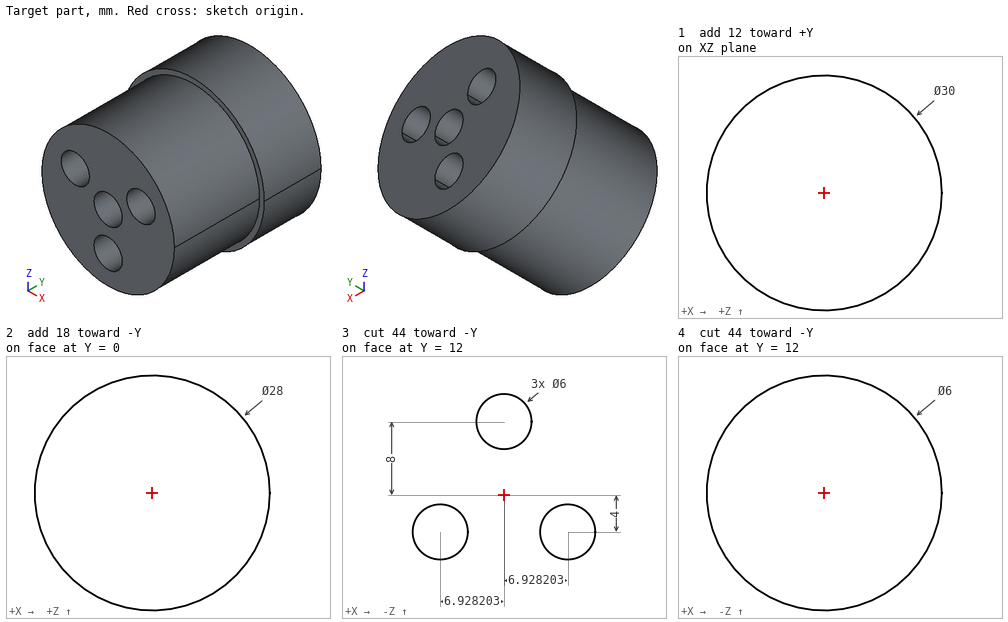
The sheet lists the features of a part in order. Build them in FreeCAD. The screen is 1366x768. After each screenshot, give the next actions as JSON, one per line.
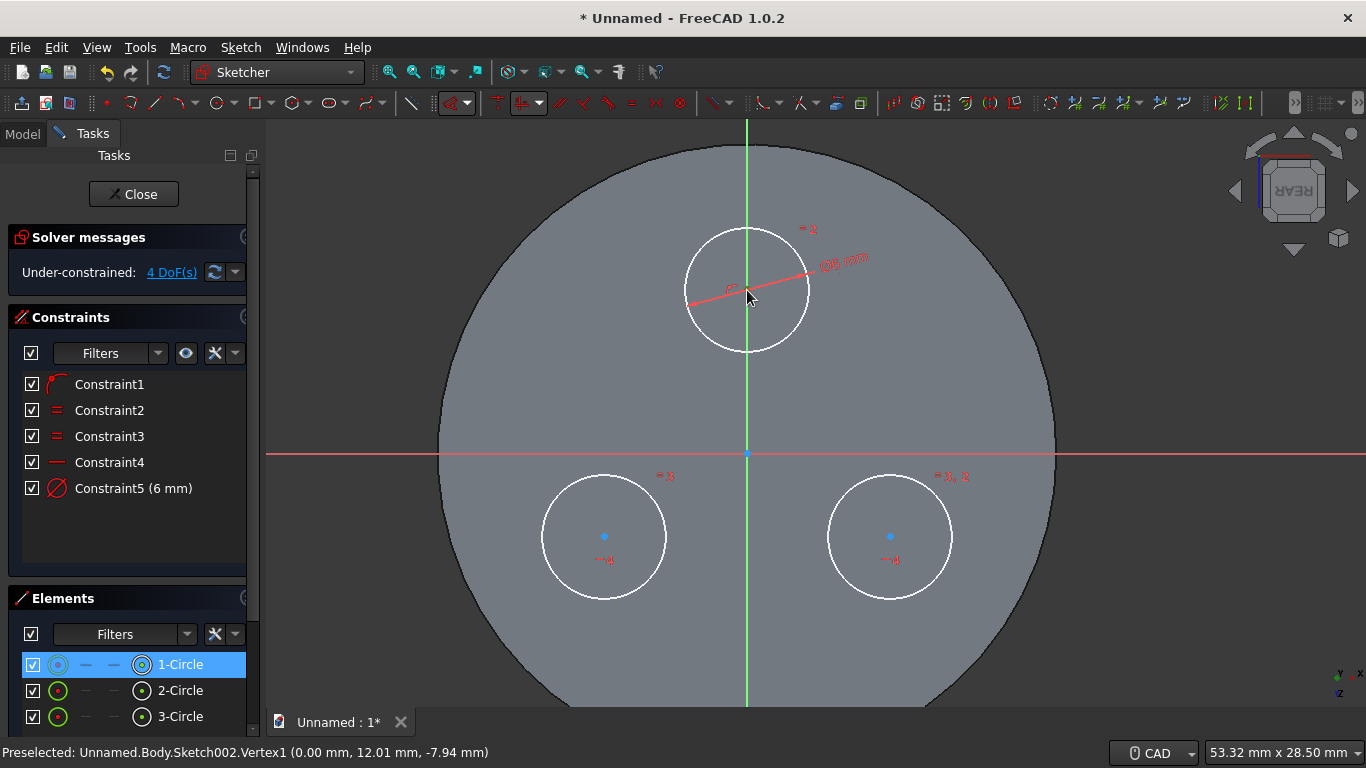
{"action": "key", "text": "i"}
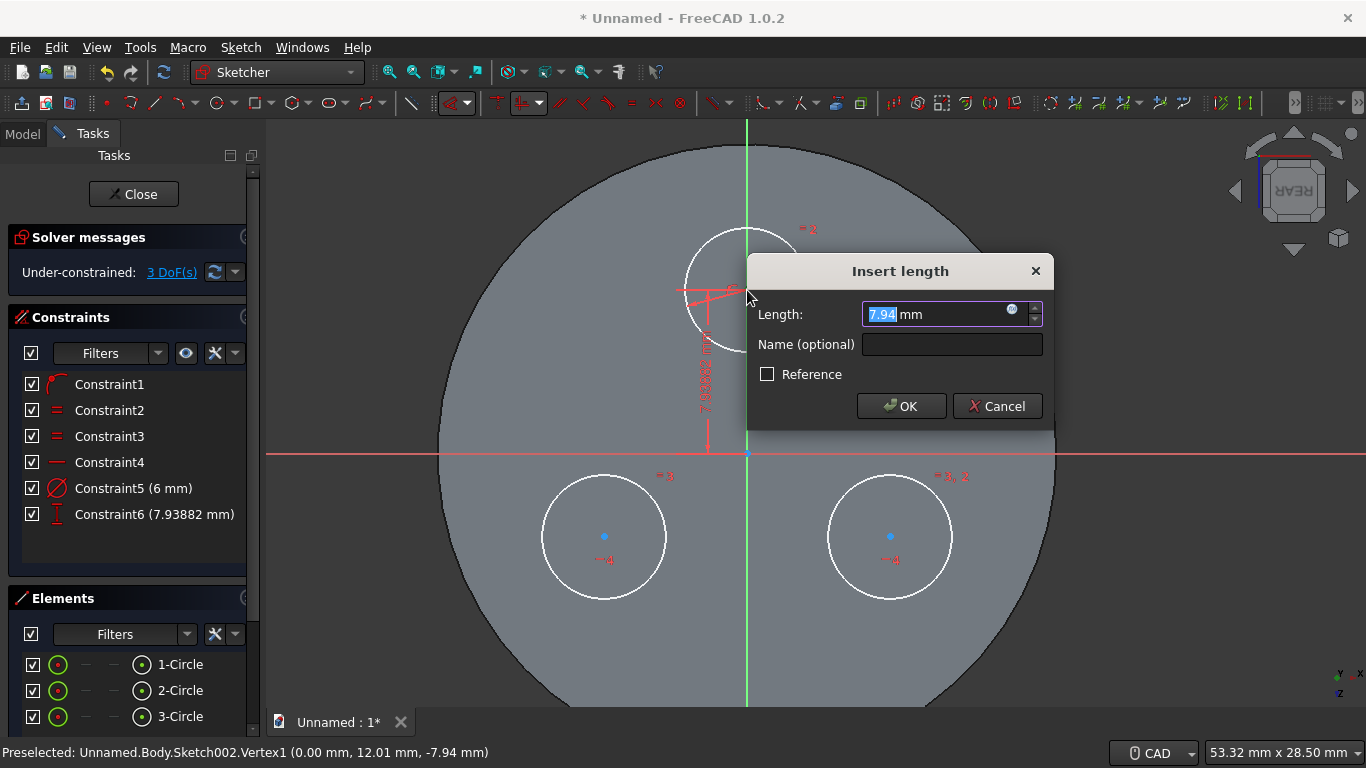
{"action": "type", "text": "8"}
{"action": "key", "text": "Return"}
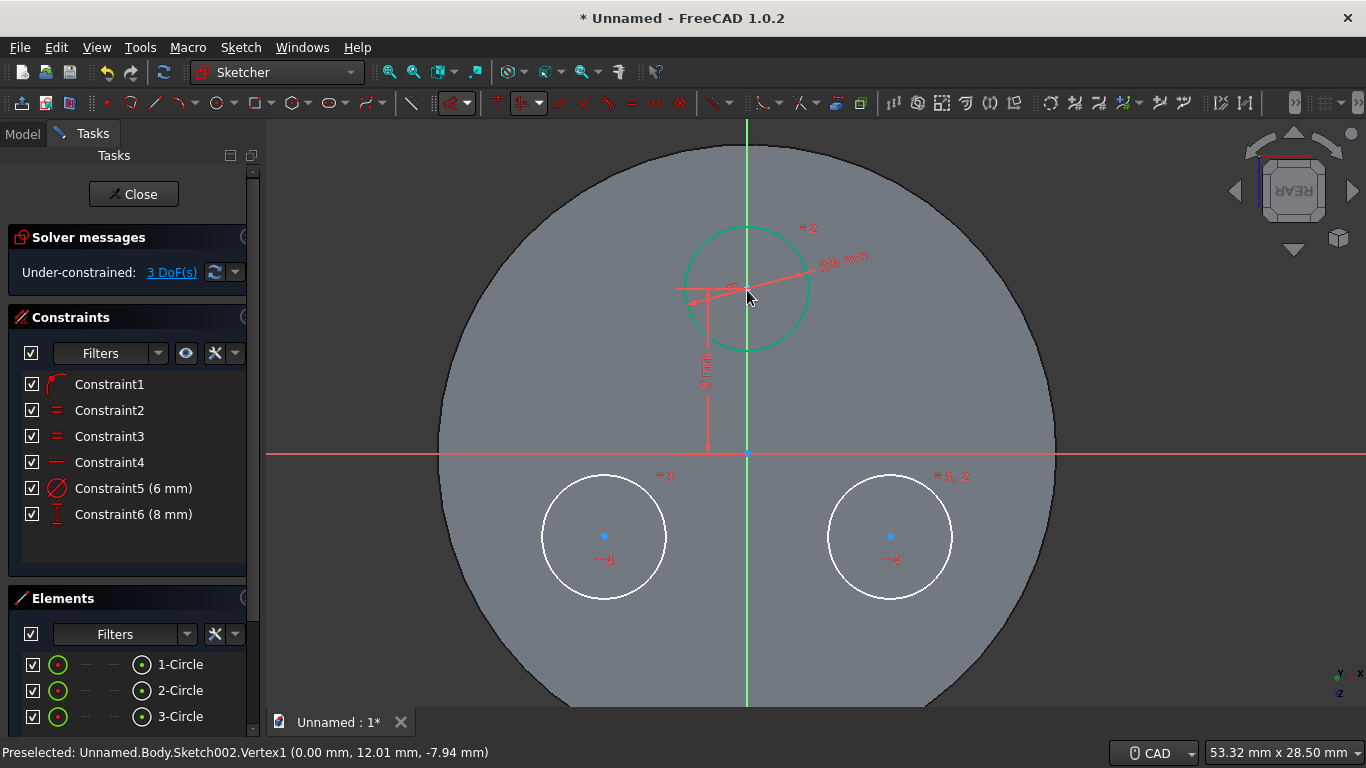
{"action": "left_click", "coordinate": [890, 537]}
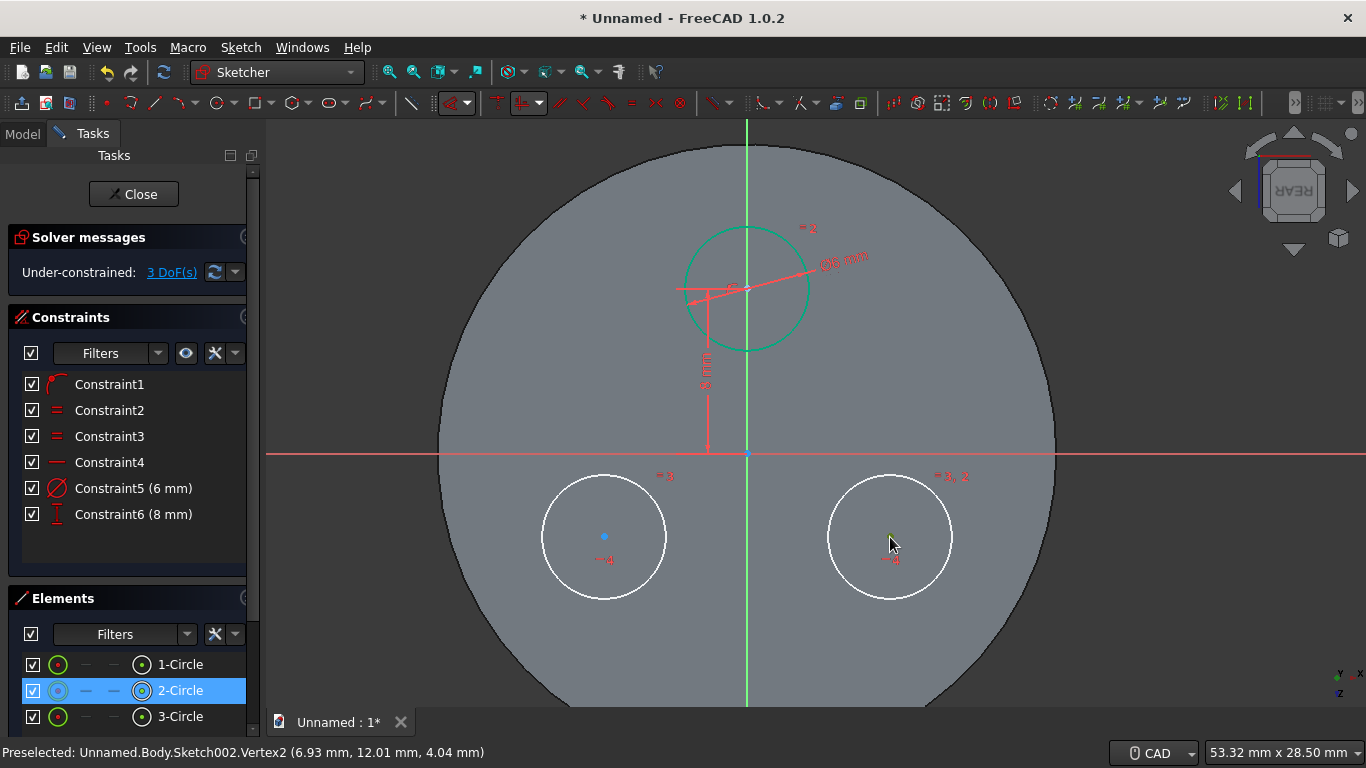
{"action": "key", "text": "i"}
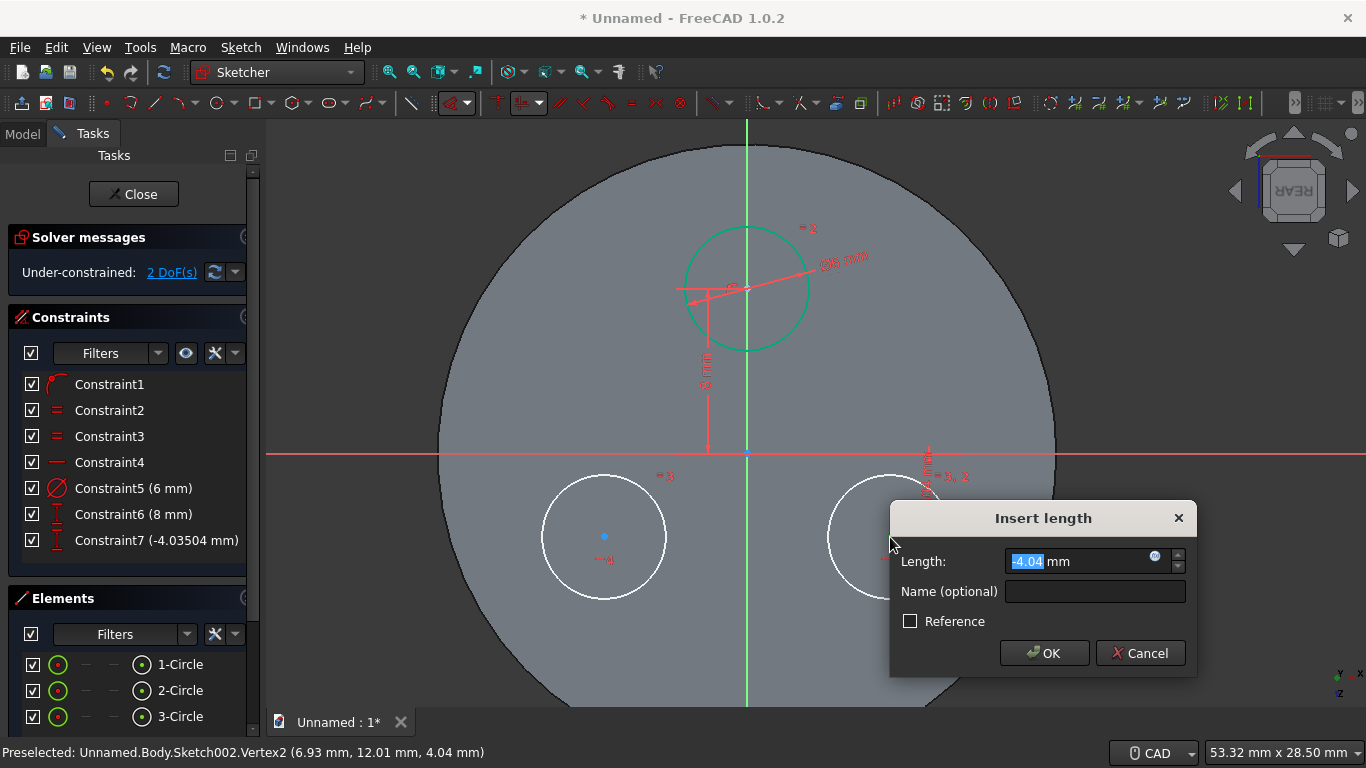
{"action": "type", "text": "-4"}
{"action": "key", "text": "Return"}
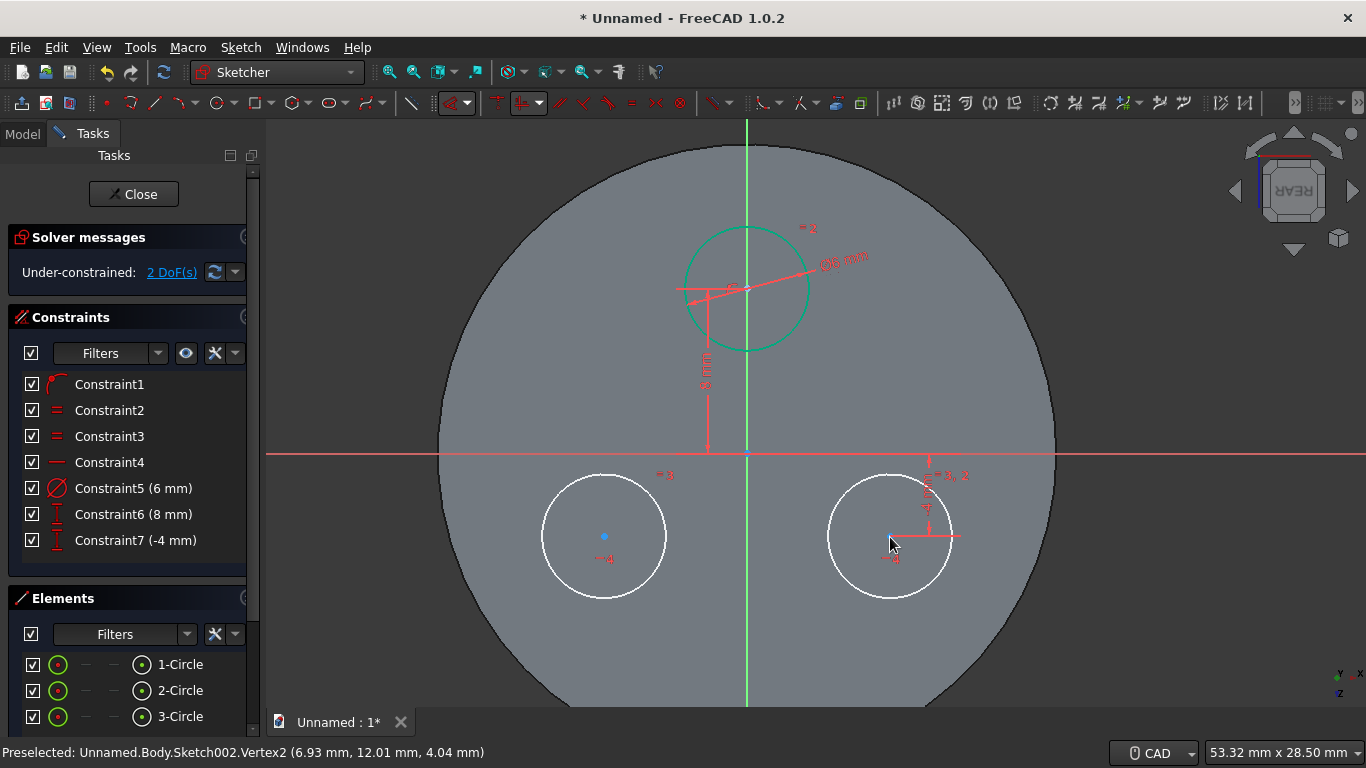
{"action": "left_click", "coordinate": [890, 536]}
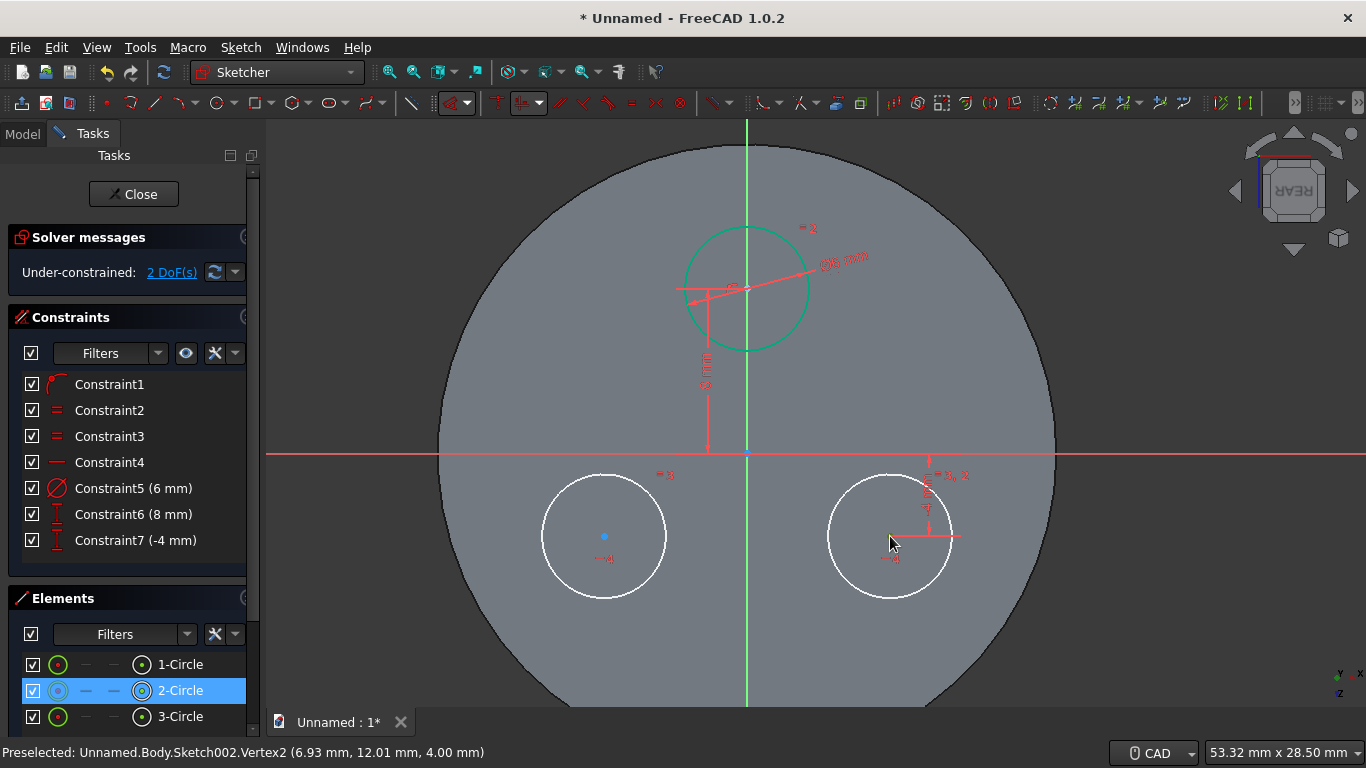
{"action": "left_click", "coordinate": [470, 104]}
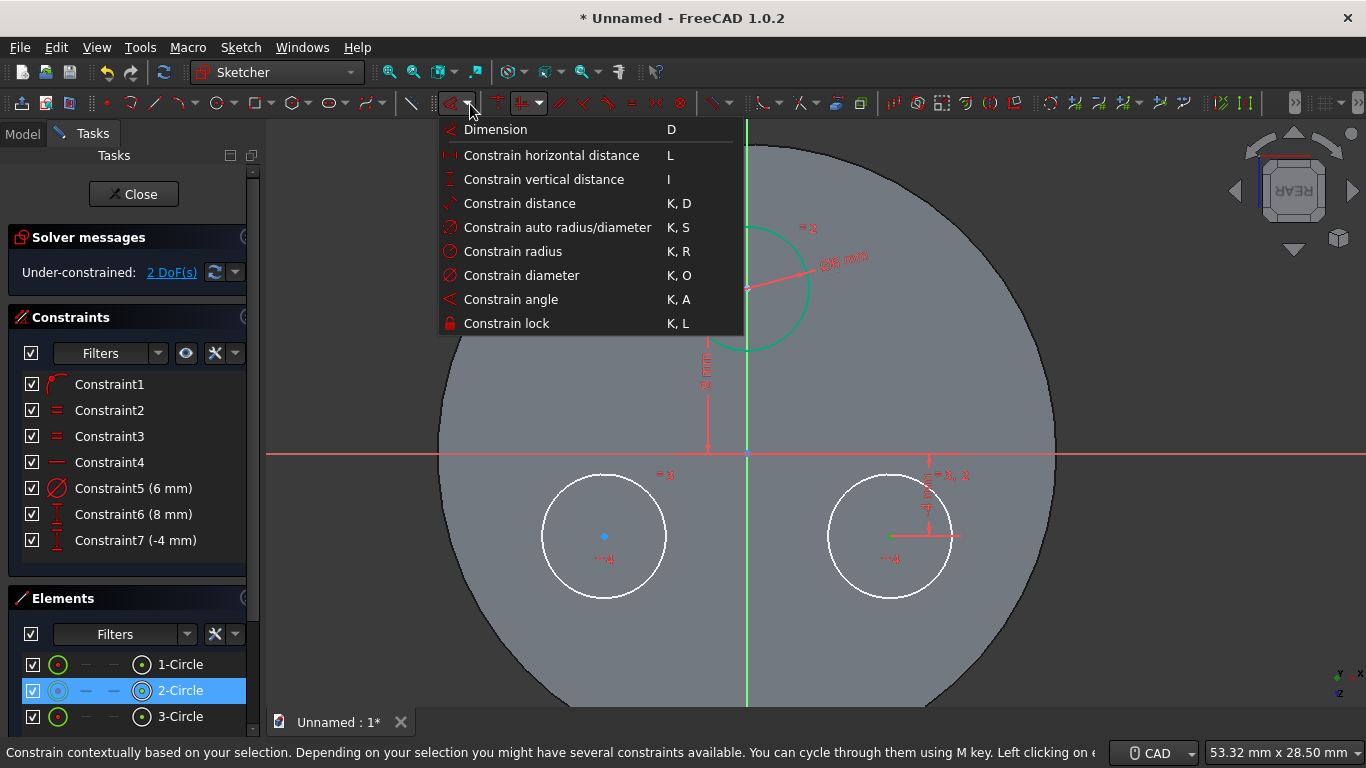
{"action": "left_click", "coordinate": [591, 155]}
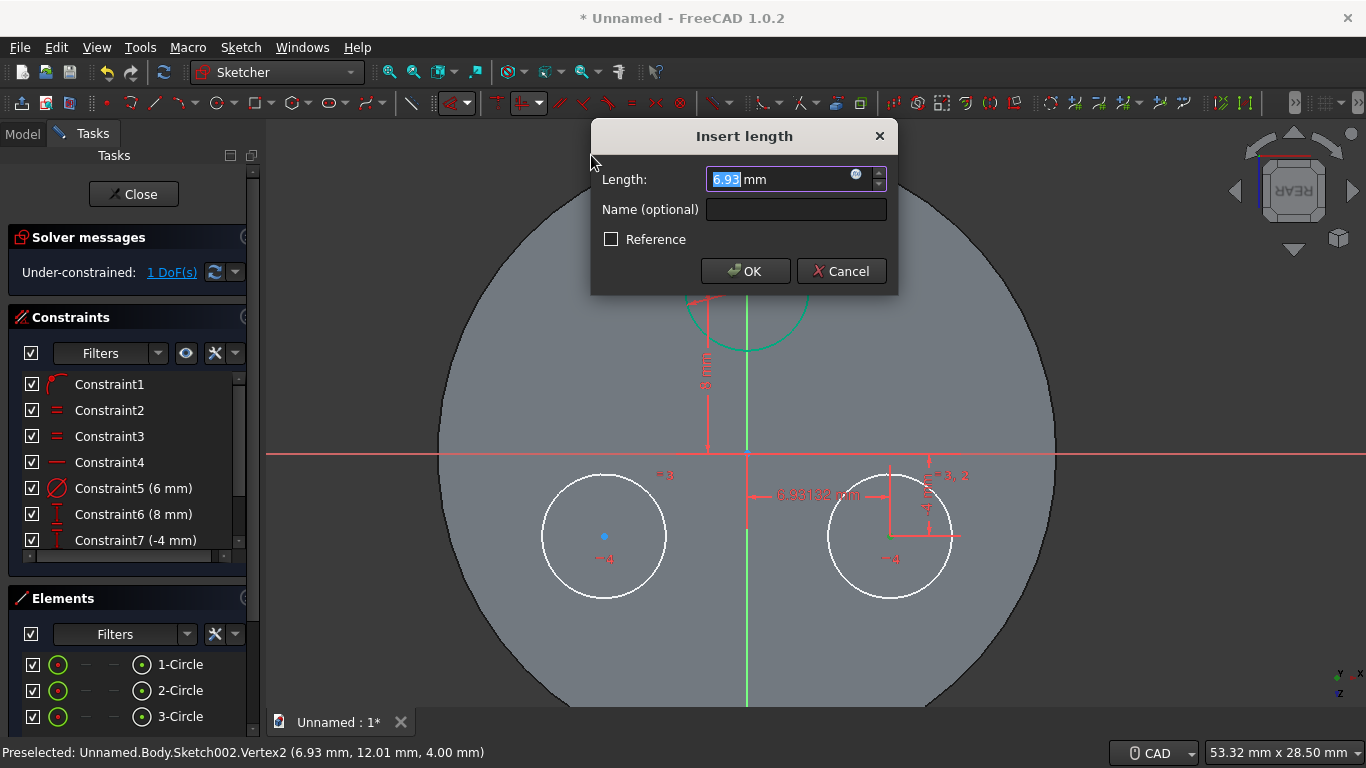
{"action": "type", "text": "6.928203"}
{"action": "key", "text": "Return"}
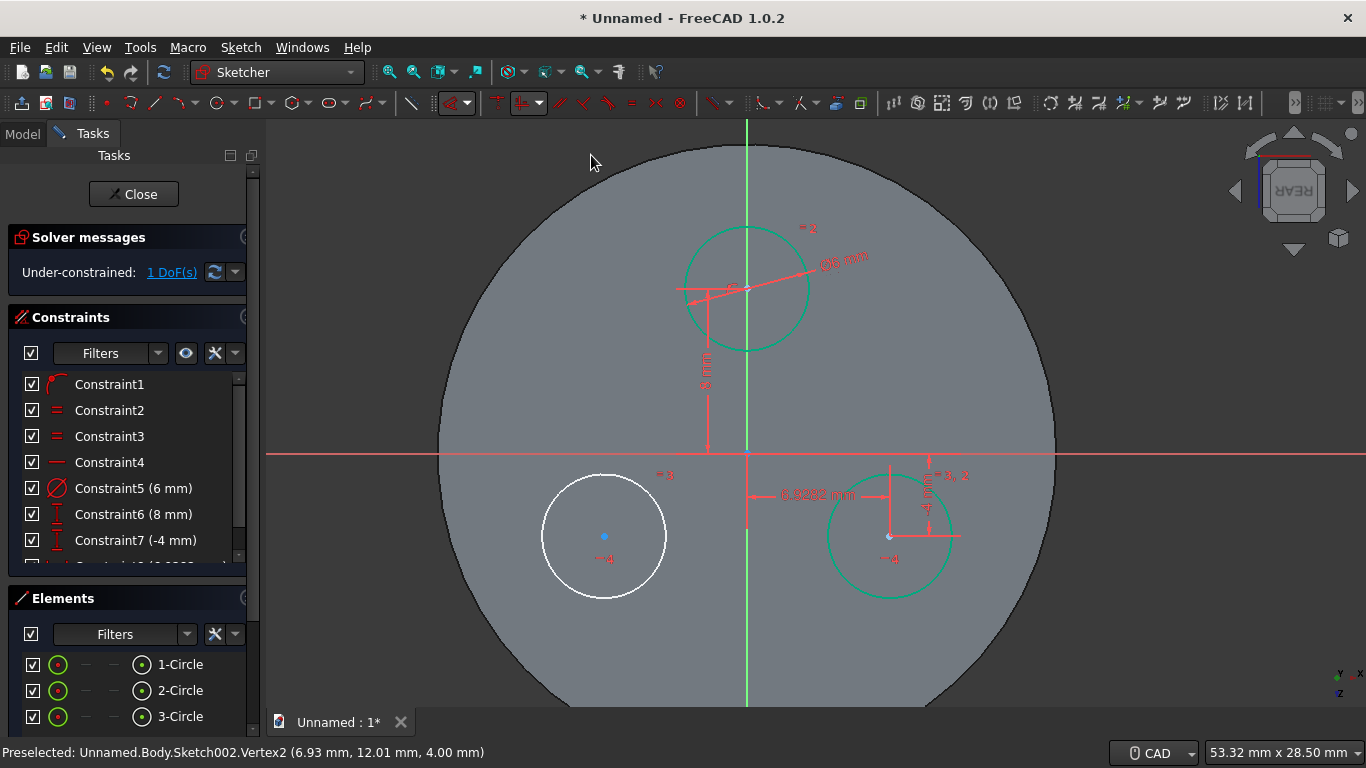
{"action": "left_click", "coordinate": [604, 536]}